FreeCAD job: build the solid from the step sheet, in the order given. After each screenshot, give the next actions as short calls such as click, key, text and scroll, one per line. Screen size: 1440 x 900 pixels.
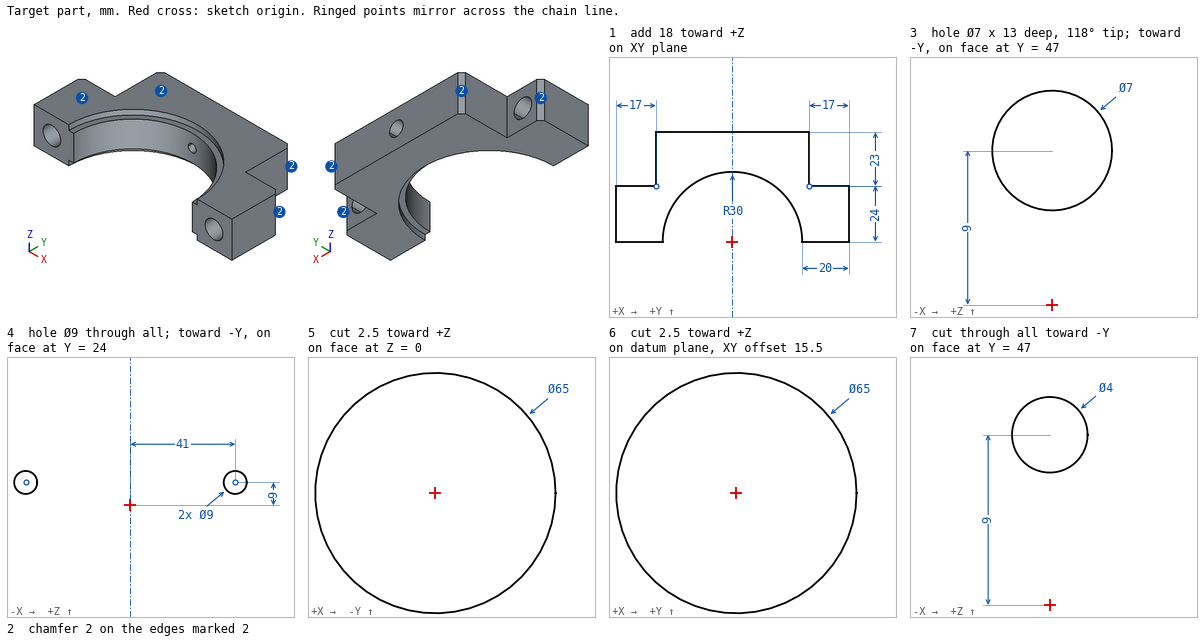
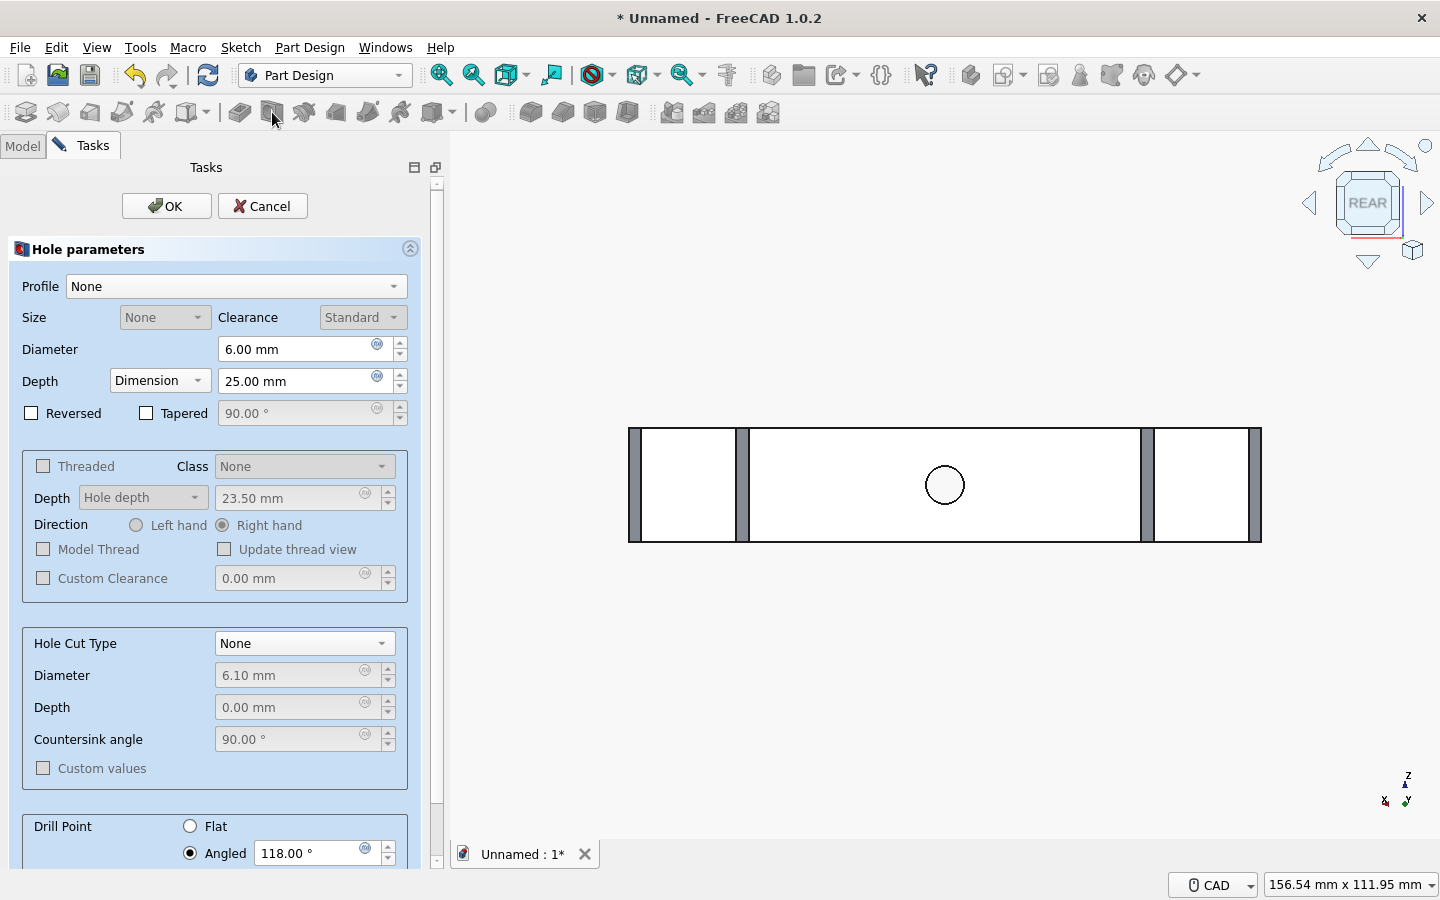
triple_click(305, 349)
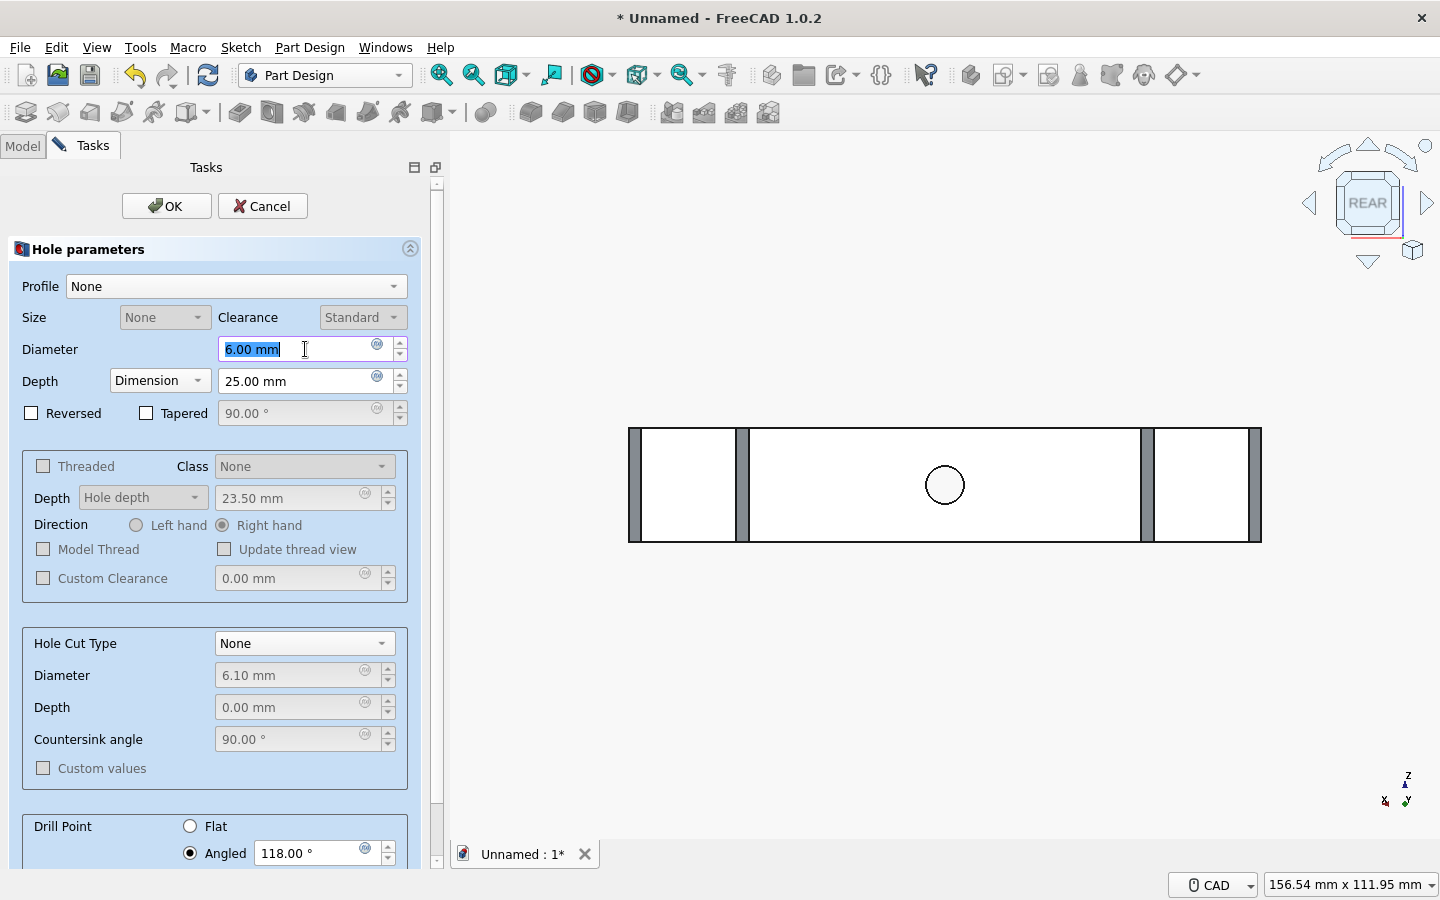
text(7)
key(Tab)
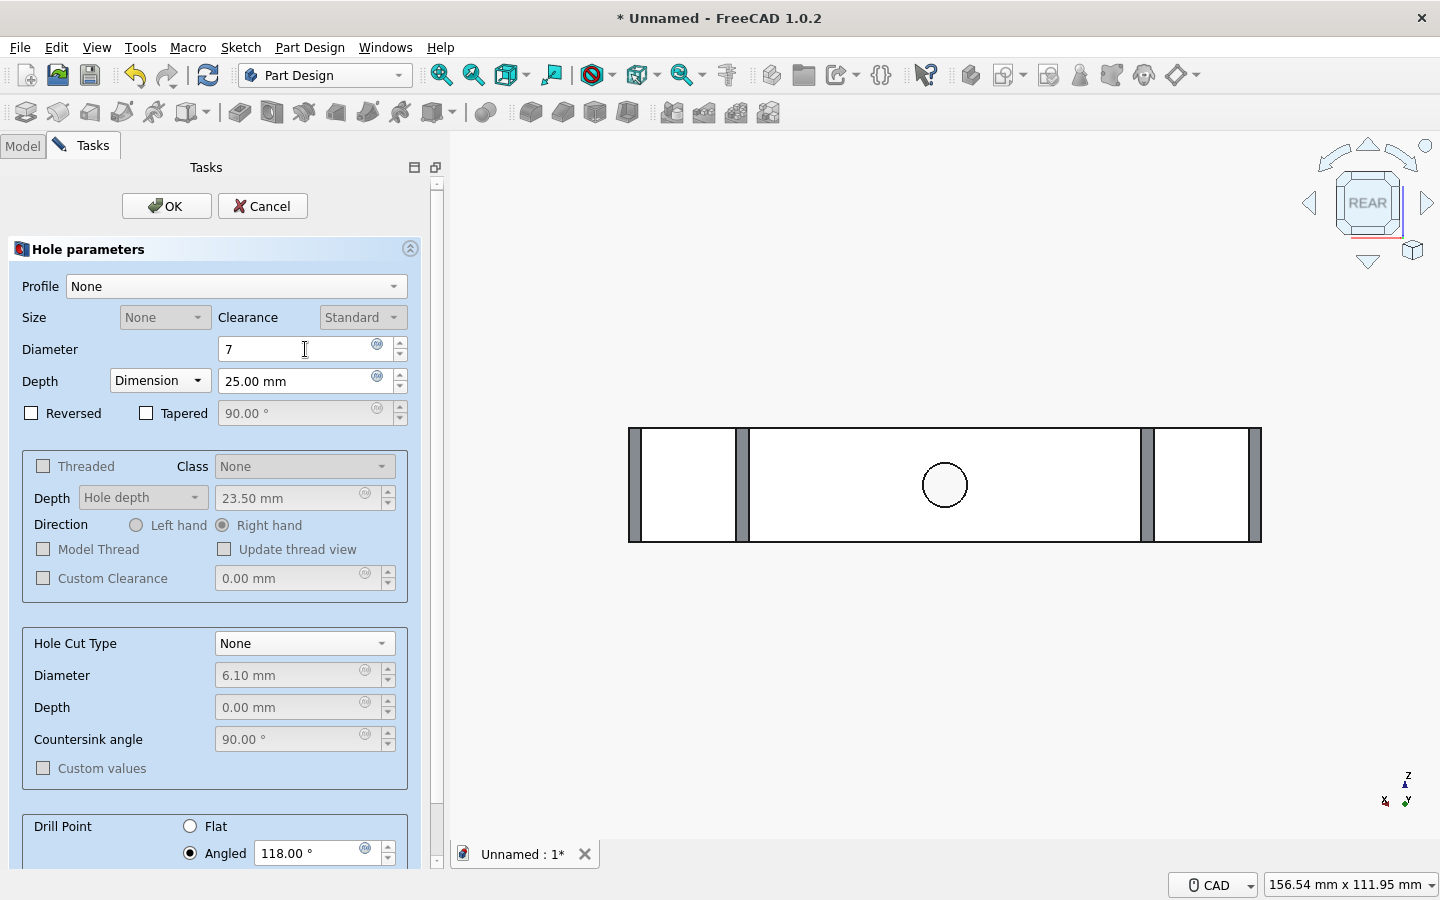
triple_click(305, 381)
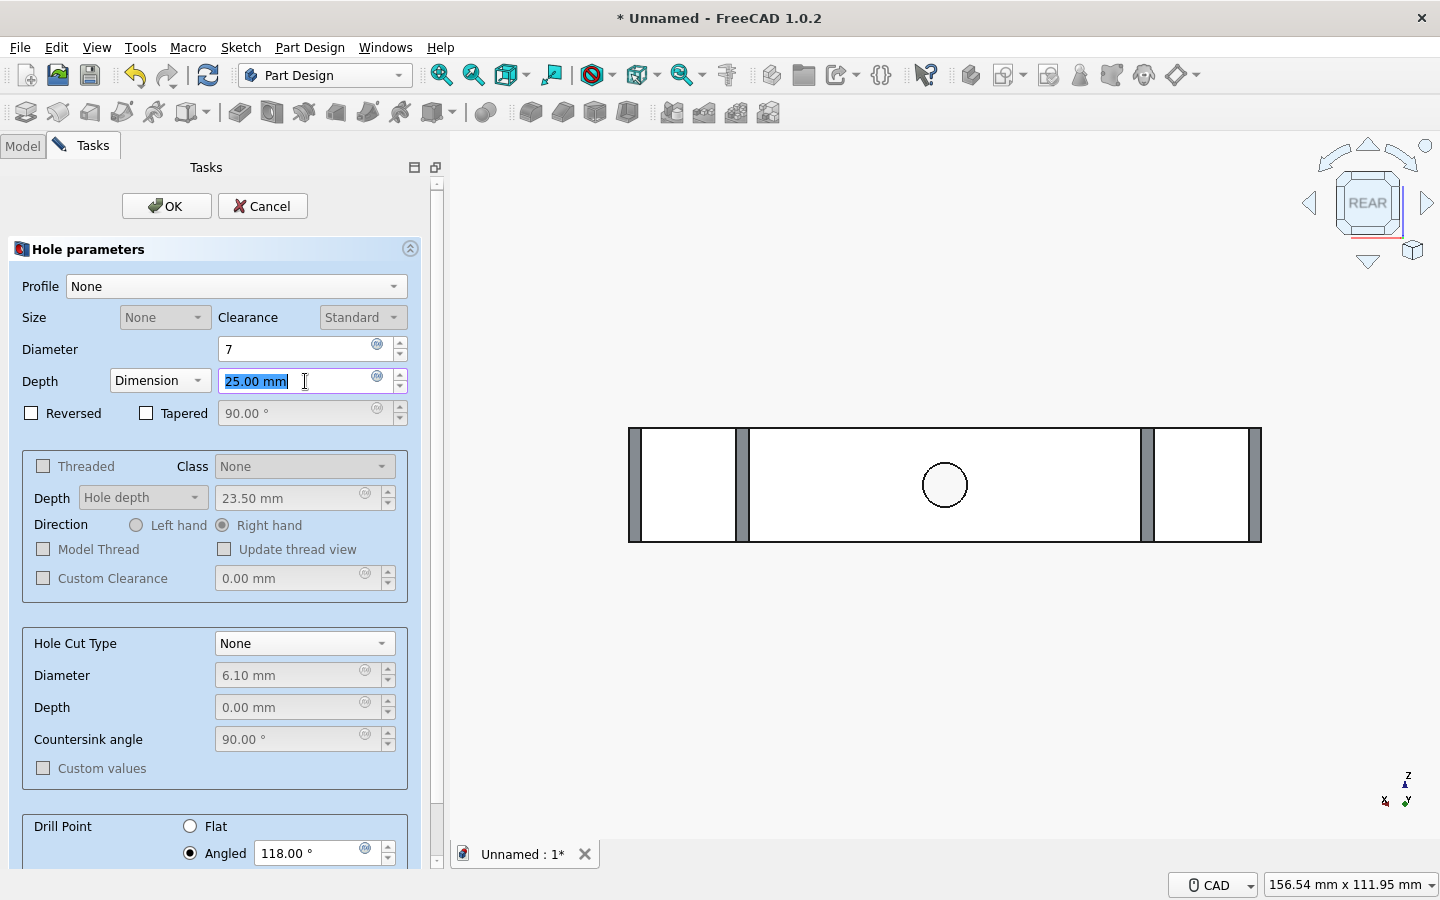
text(13)
key(Tab)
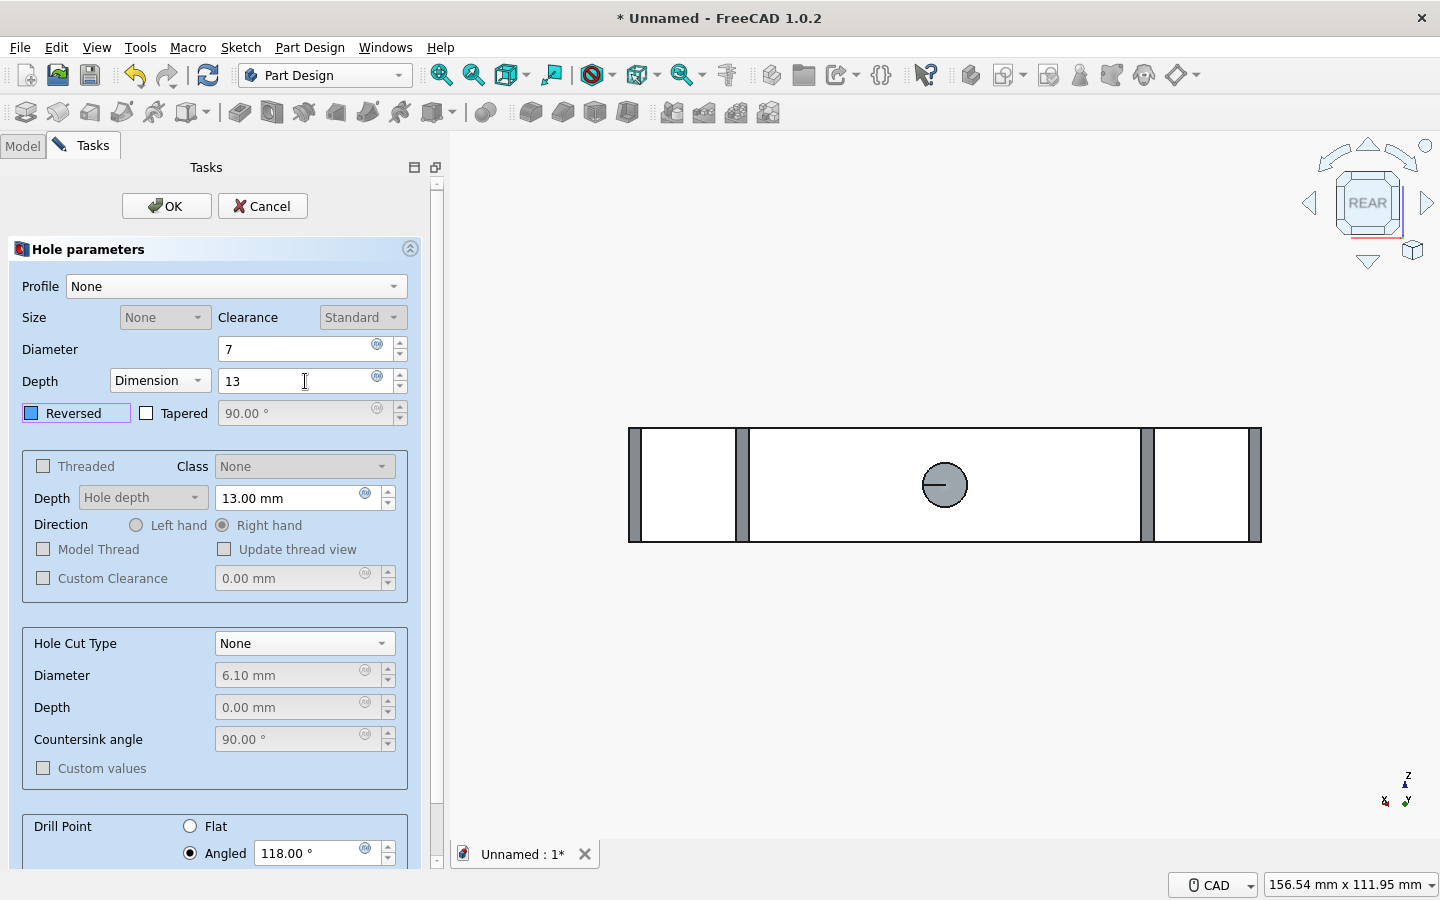
click(167, 206)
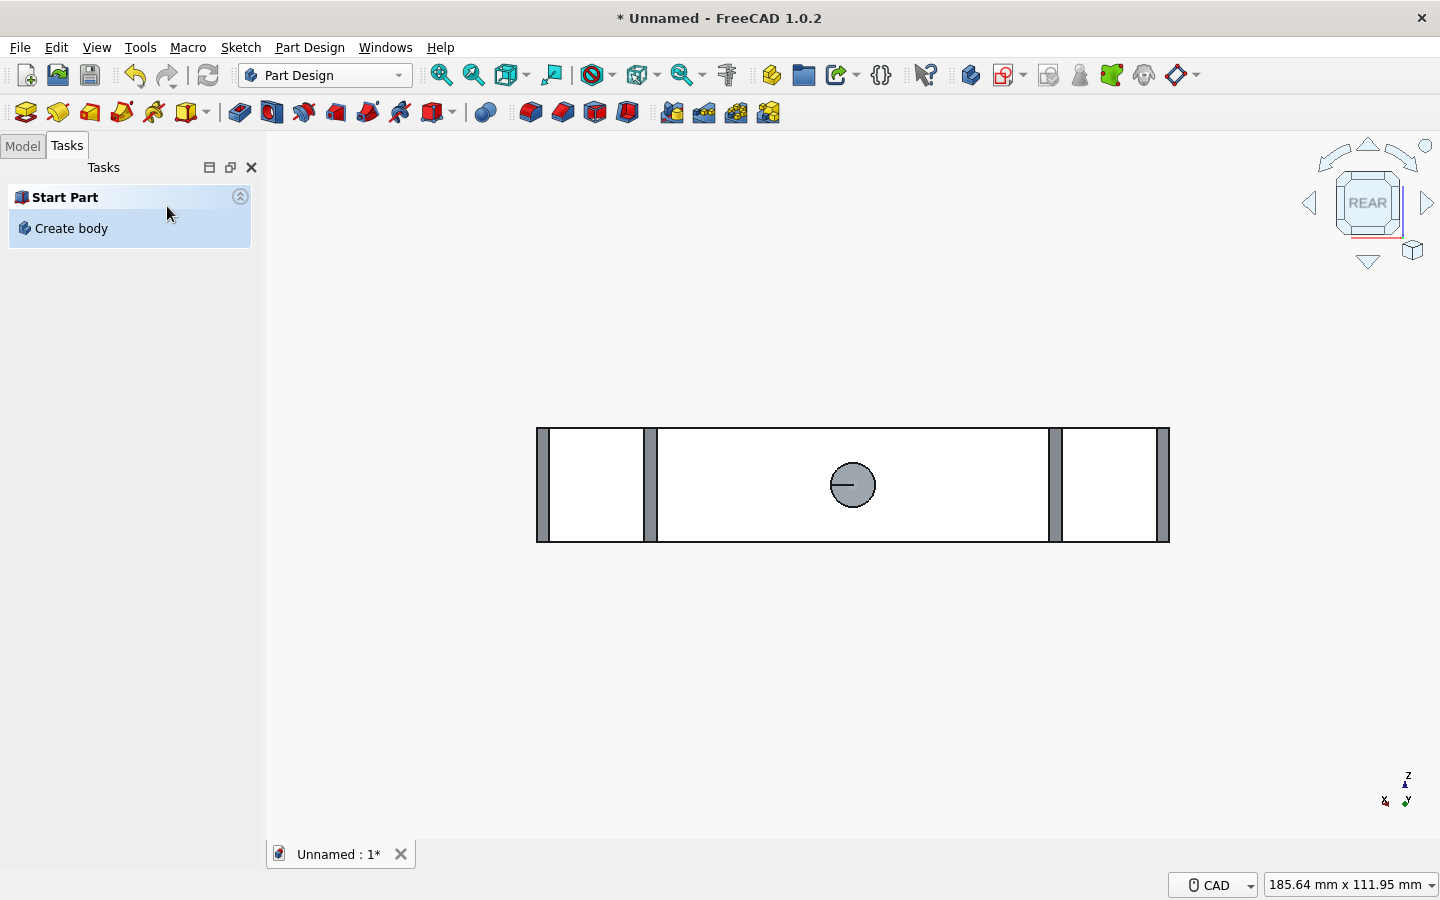
click(597, 484)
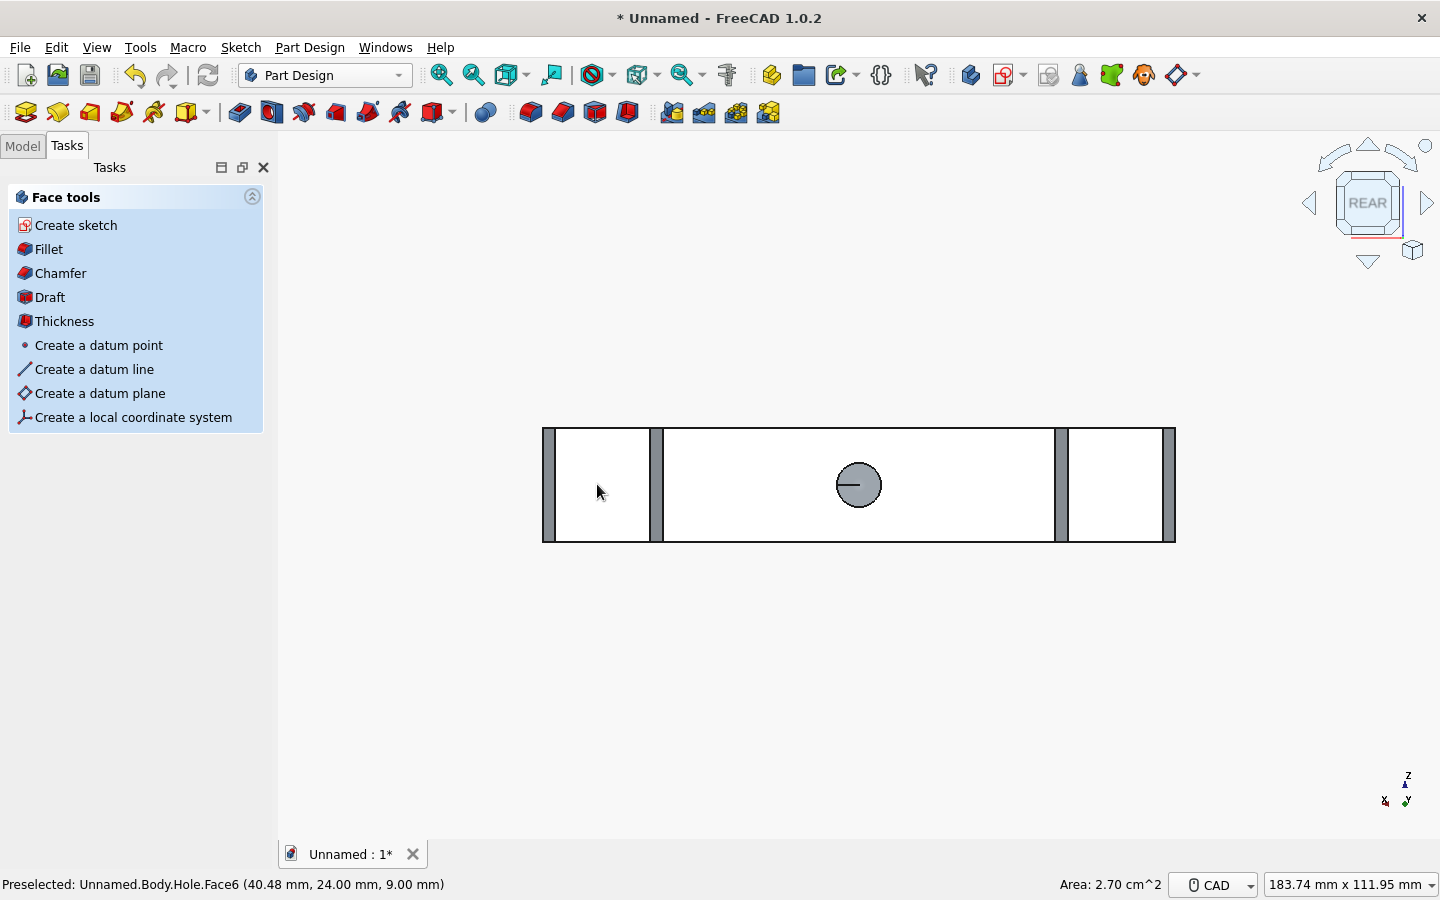
click(1004, 76)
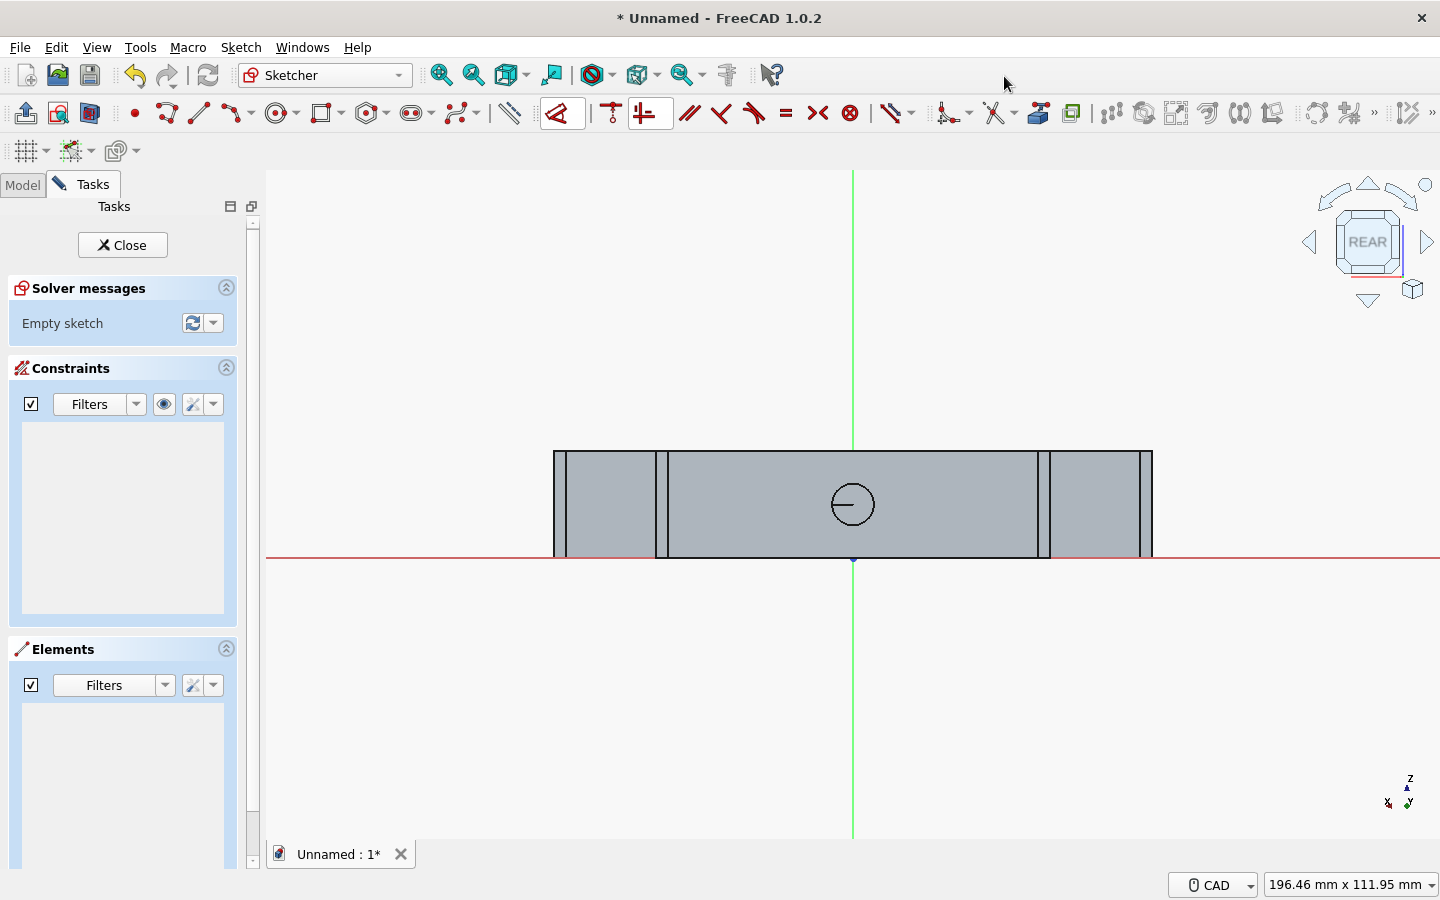
click(90, 114)